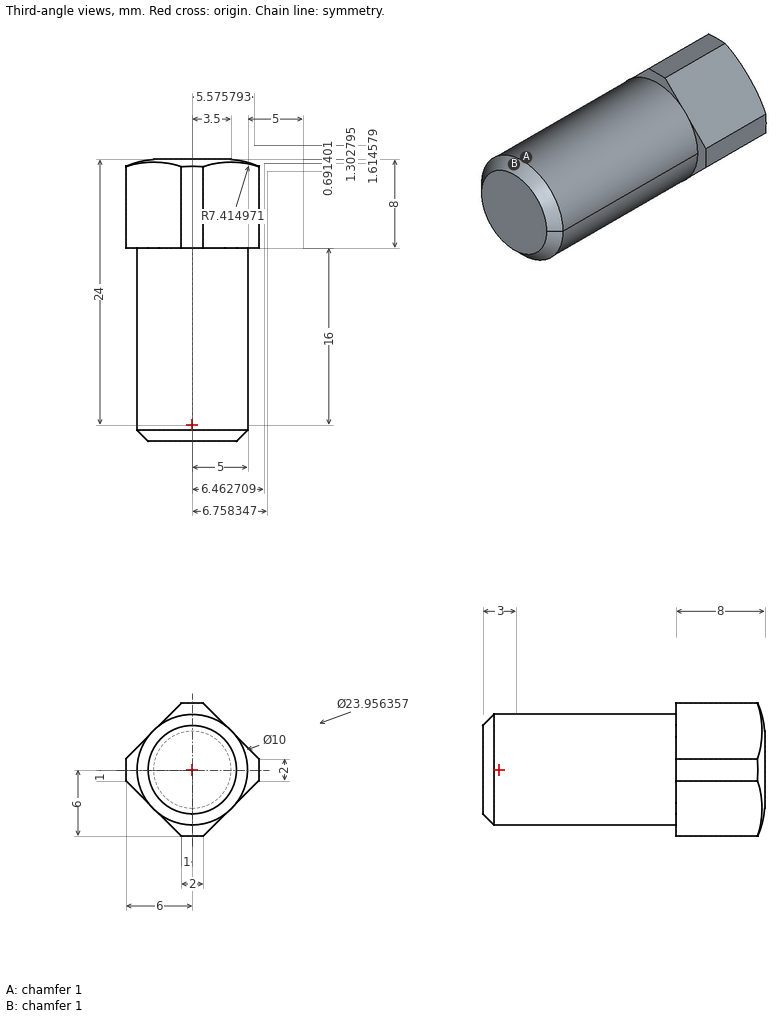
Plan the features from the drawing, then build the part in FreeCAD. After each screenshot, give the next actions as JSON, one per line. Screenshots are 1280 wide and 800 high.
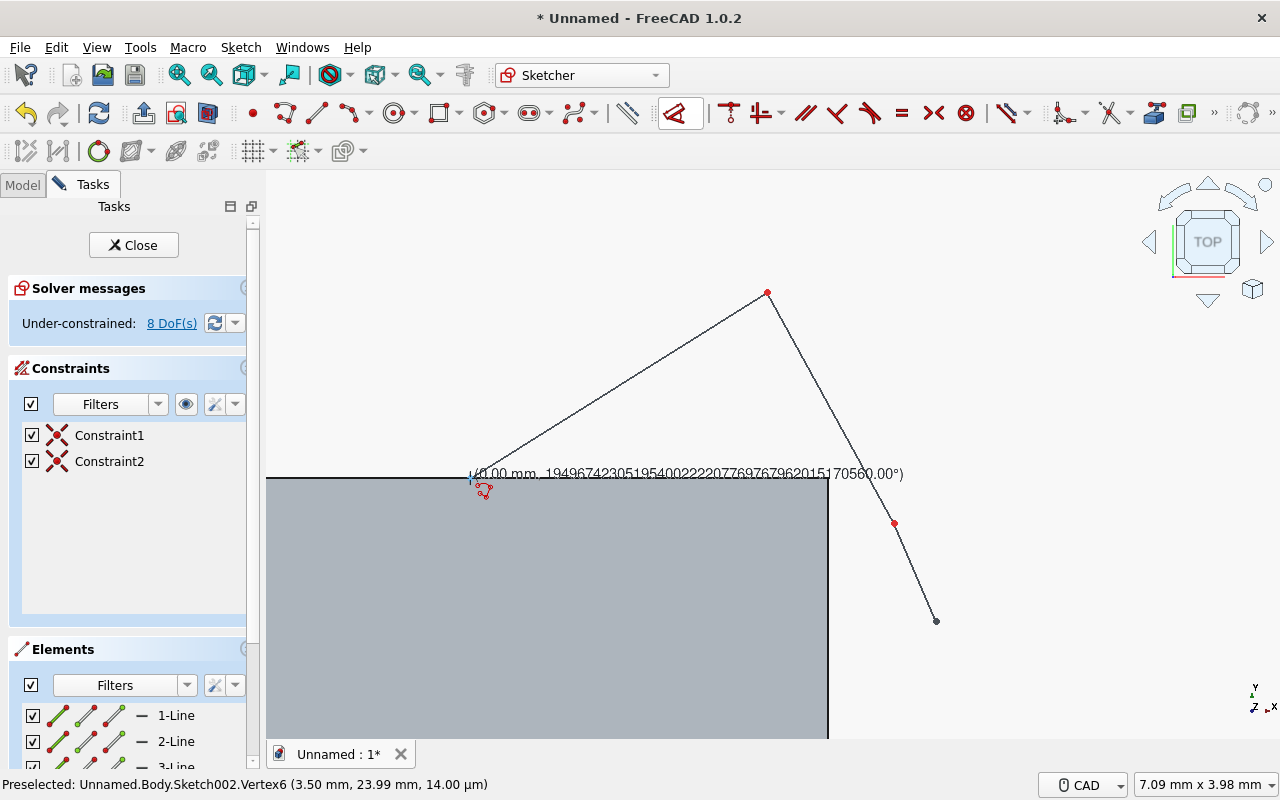
{"action": "left_click", "coordinate": [350, 114]}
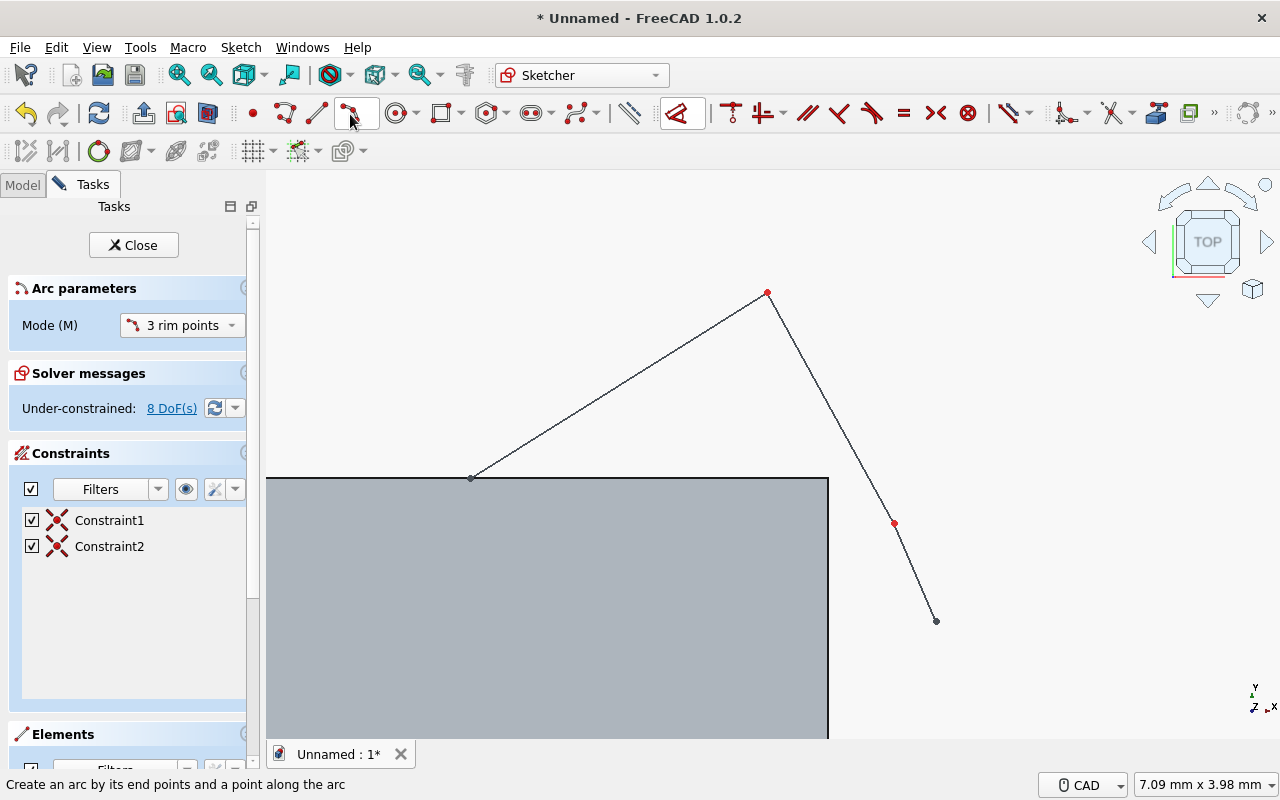
{"action": "left_click", "coordinate": [470, 479]}
{"action": "left_click", "coordinate": [936, 622]}
{"action": "left_click", "coordinate": [711, 523]}
{"action": "key", "text": "Escape"}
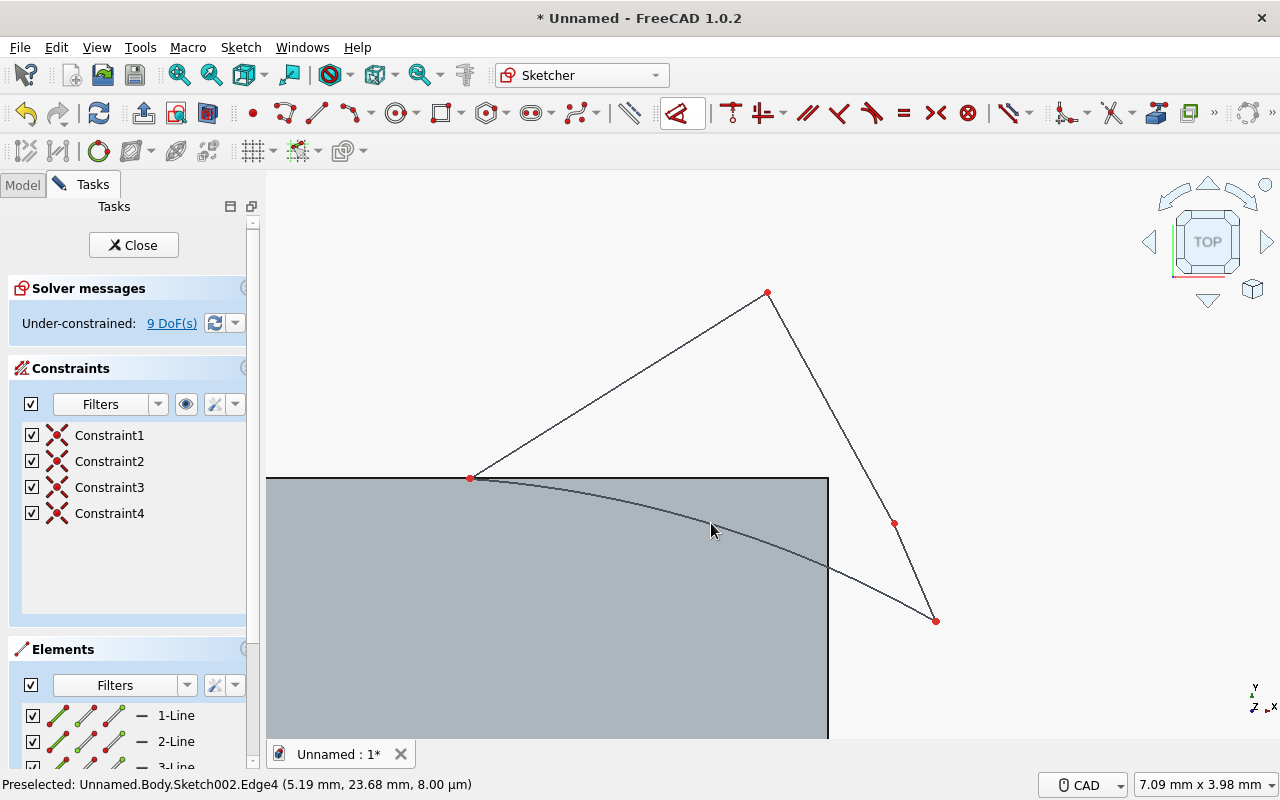
{"action": "left_click", "coordinate": [804, 557]}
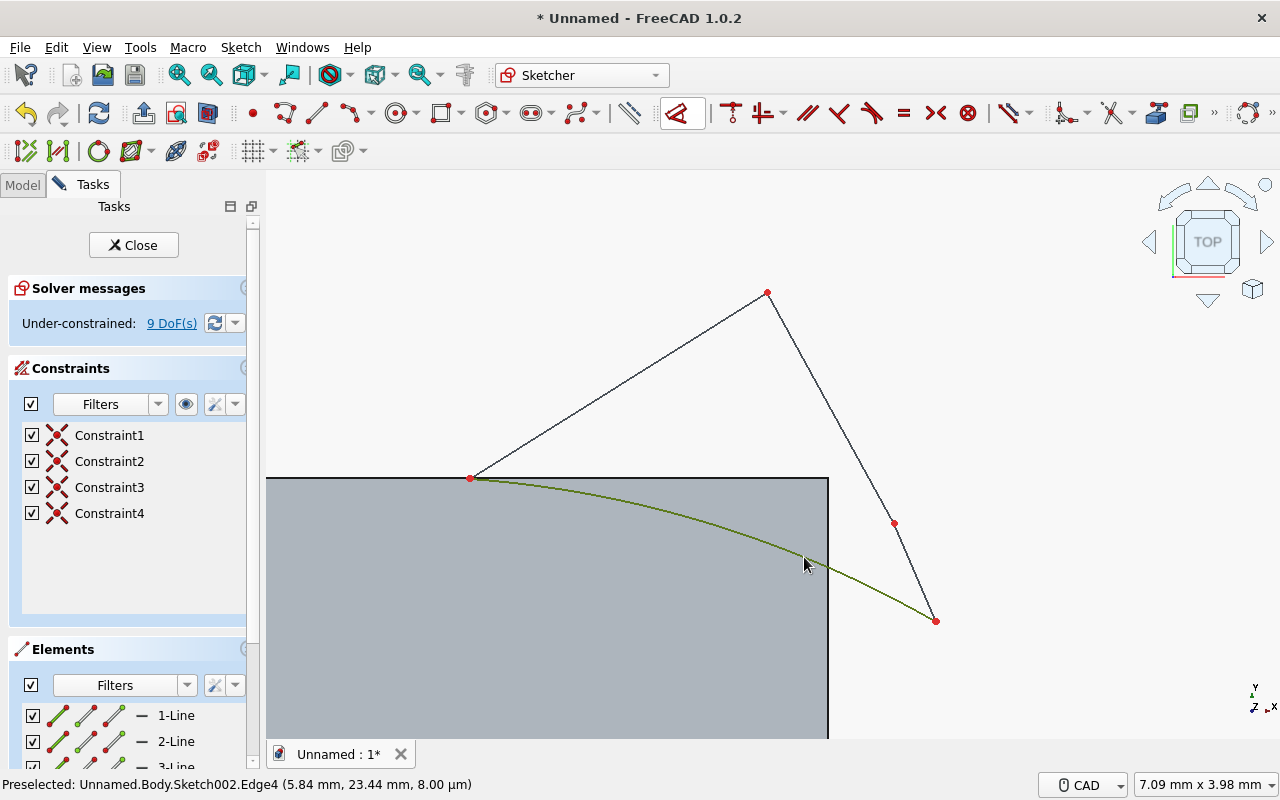
{"action": "left_click", "coordinate": [700, 114]}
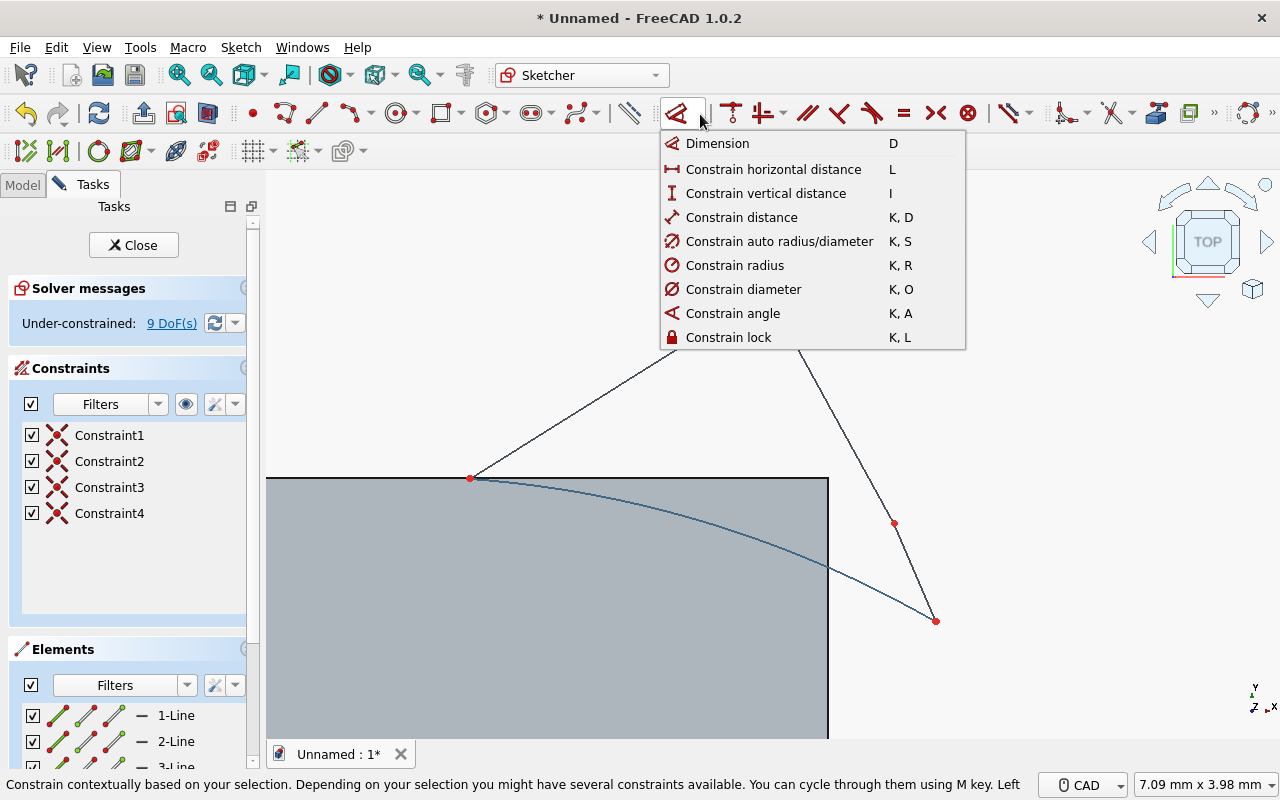
{"action": "left_click", "coordinate": [813, 265]}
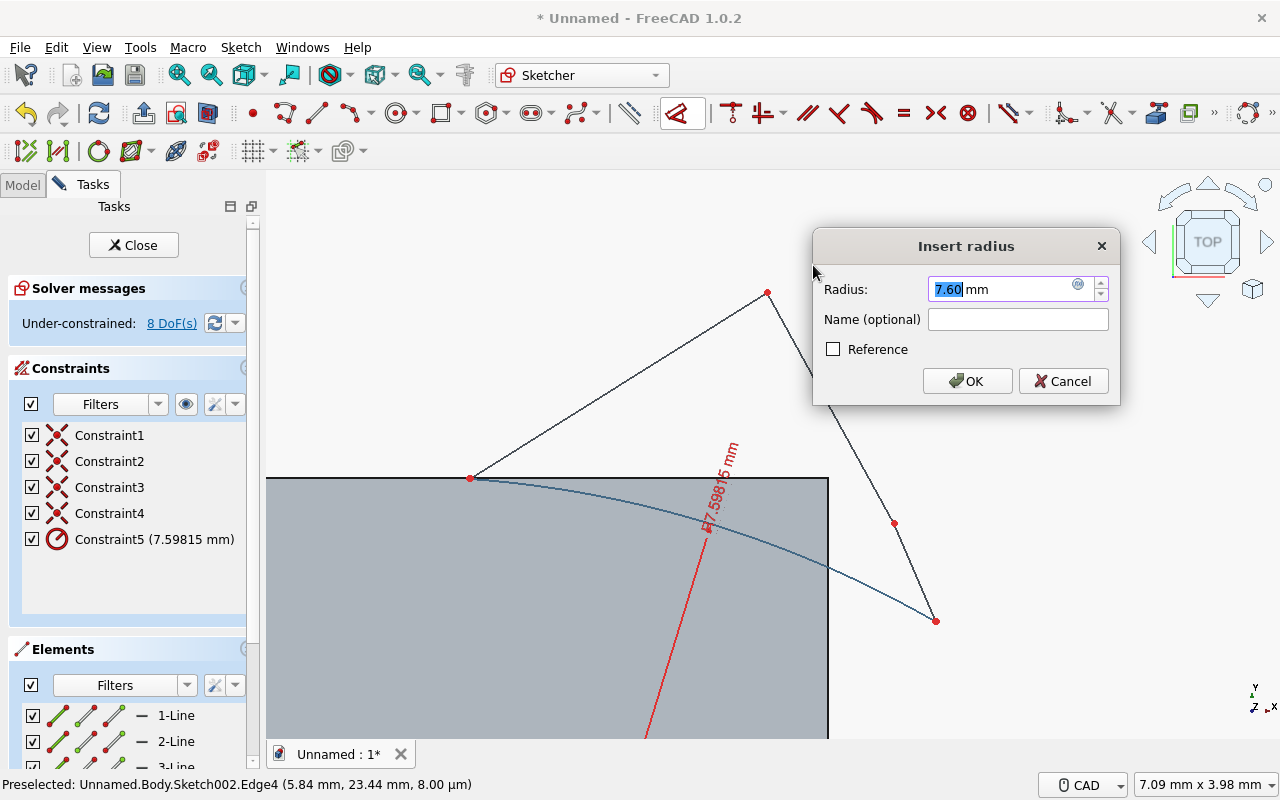
{"action": "type", "text": "7.414971"}
{"action": "key", "text": "Return"}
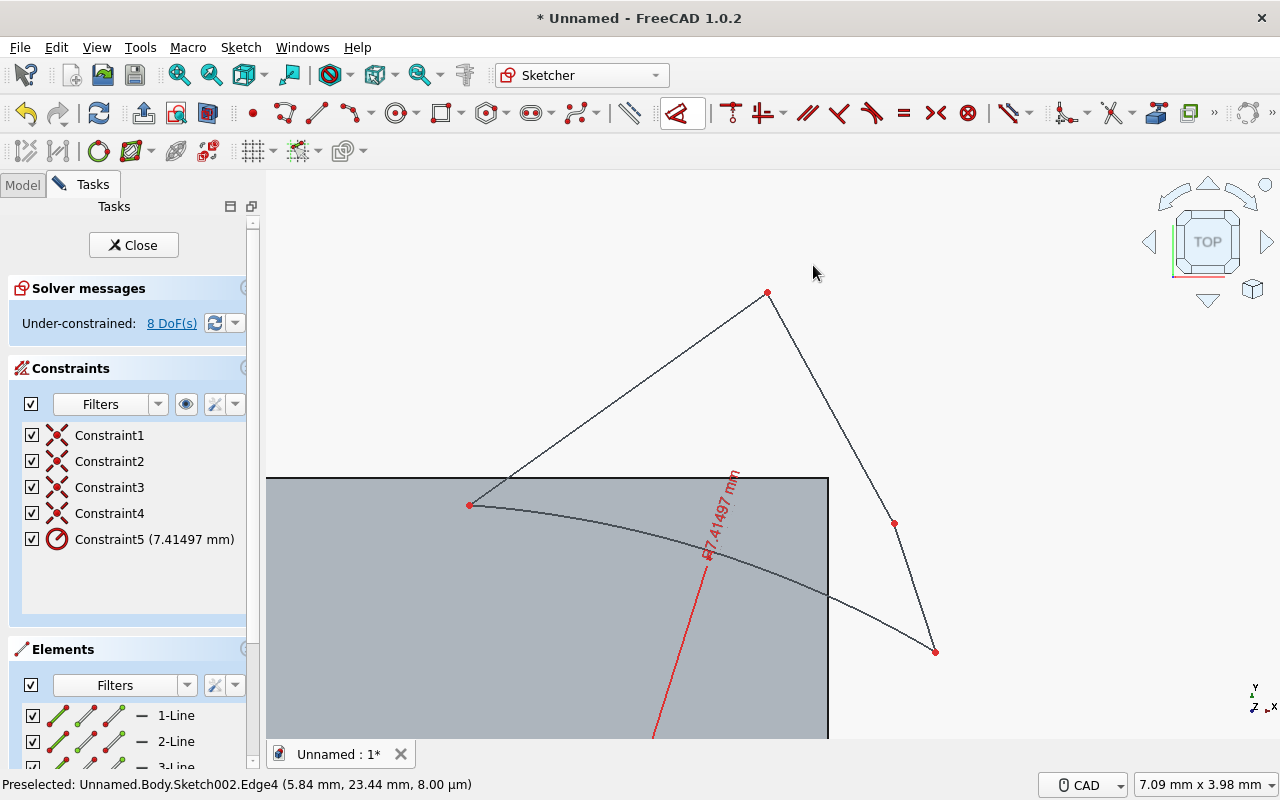
{"action": "left_click", "coordinate": [470, 505]}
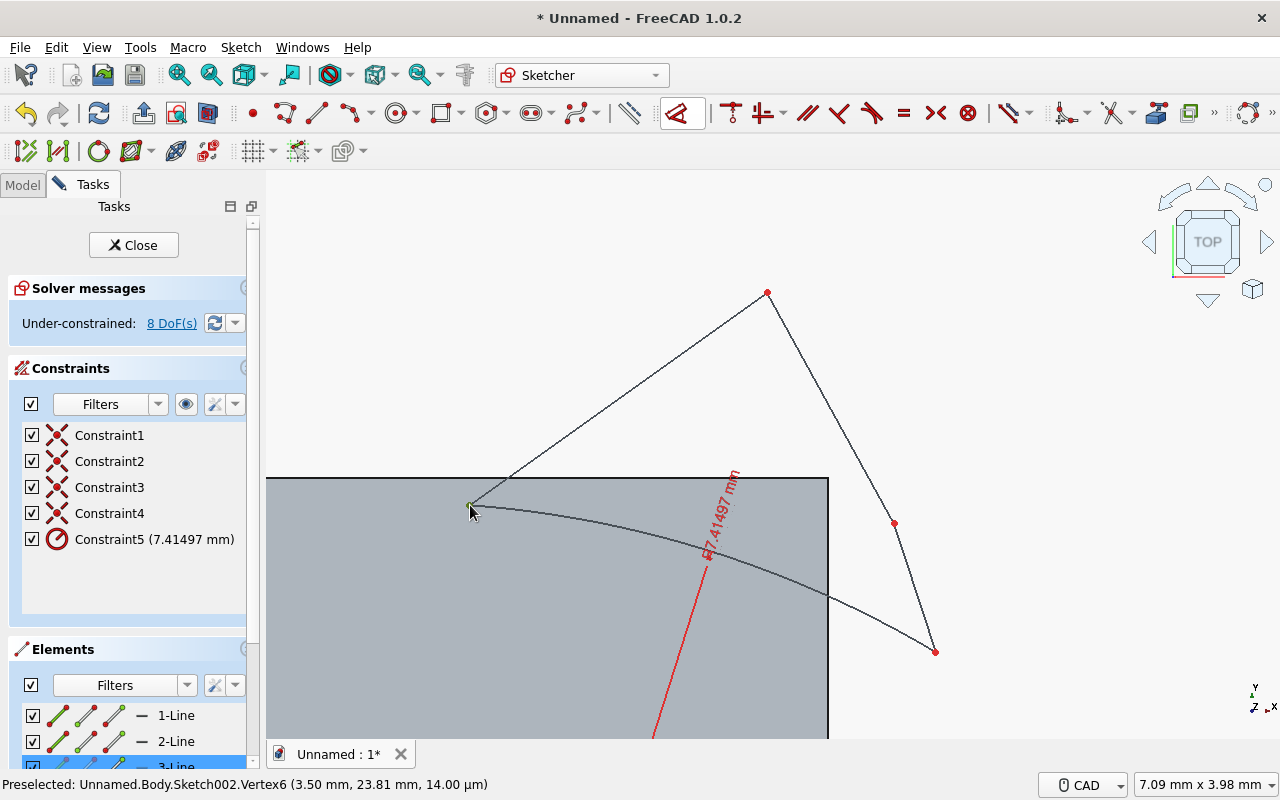
{"action": "left_click", "coordinate": [700, 114]}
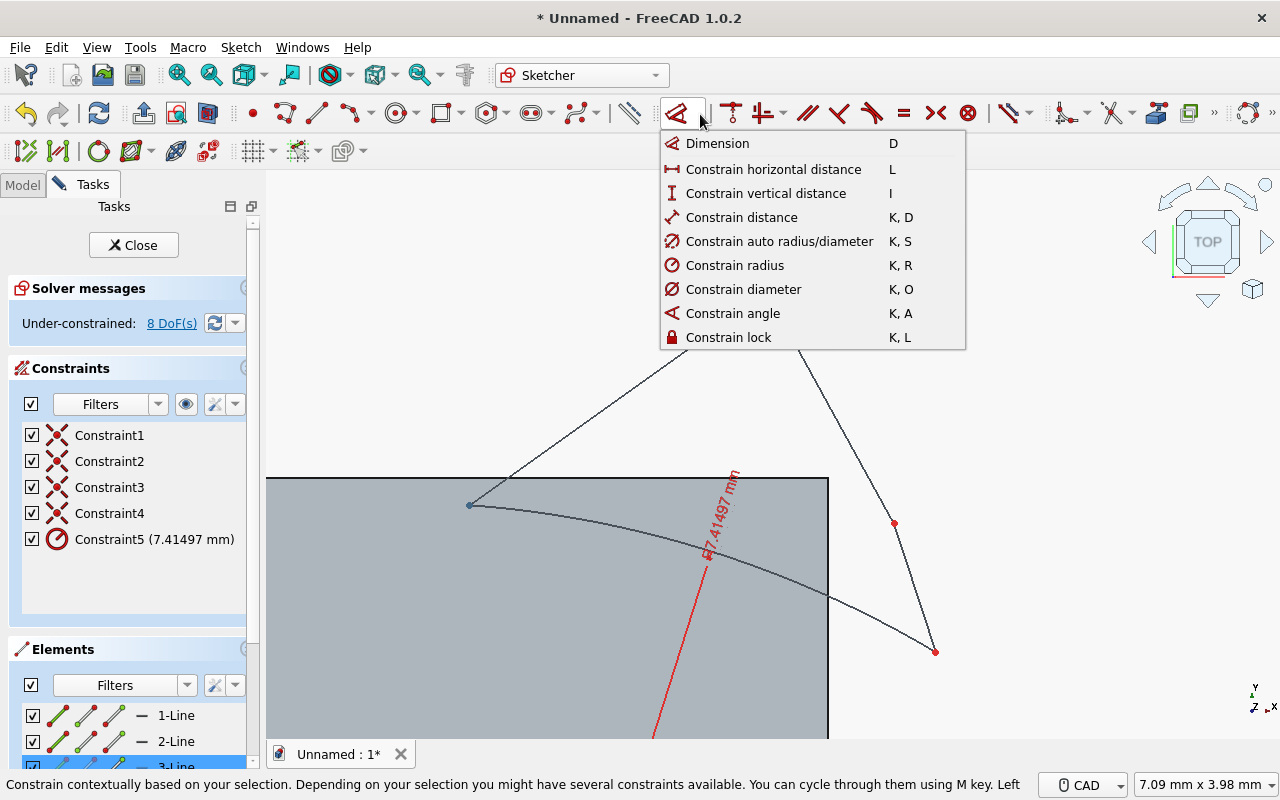
{"action": "left_click", "coordinate": [813, 193]}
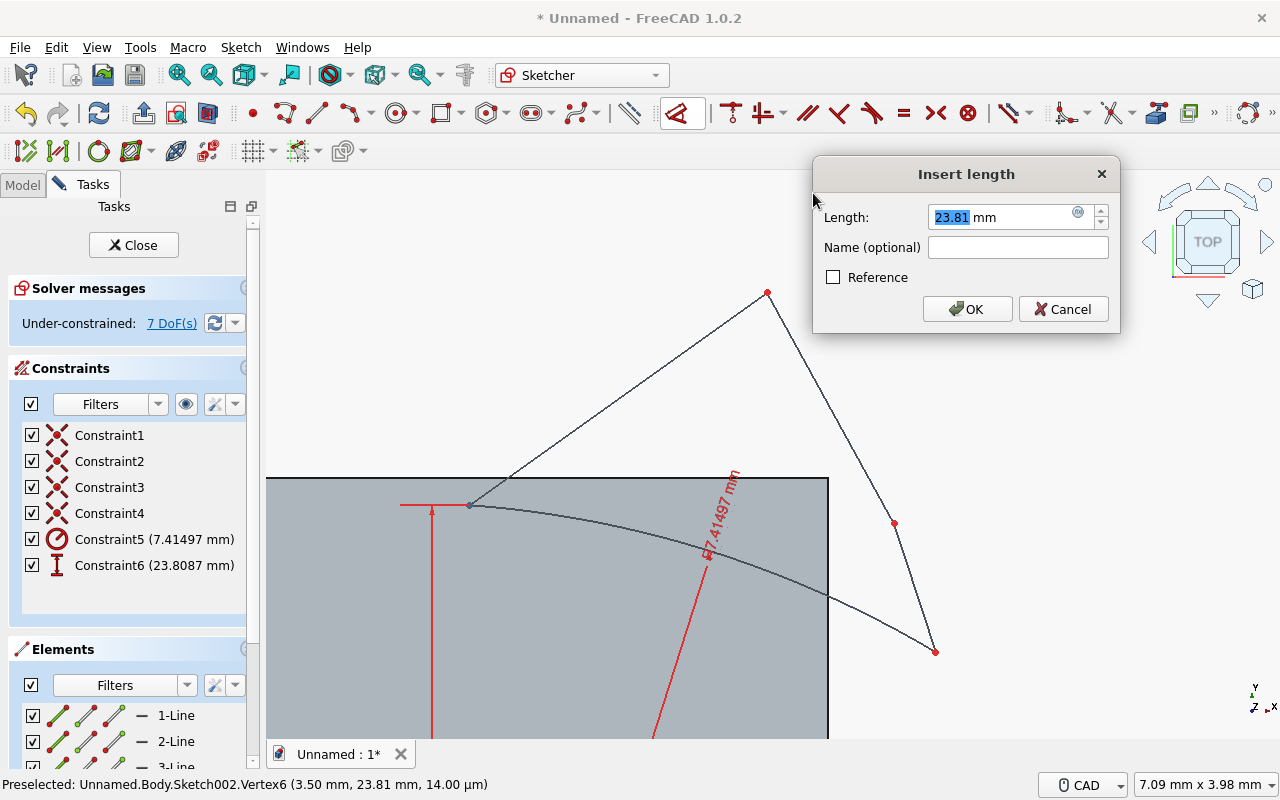
{"action": "type", "text": "24"}
{"action": "key", "text": "Return"}